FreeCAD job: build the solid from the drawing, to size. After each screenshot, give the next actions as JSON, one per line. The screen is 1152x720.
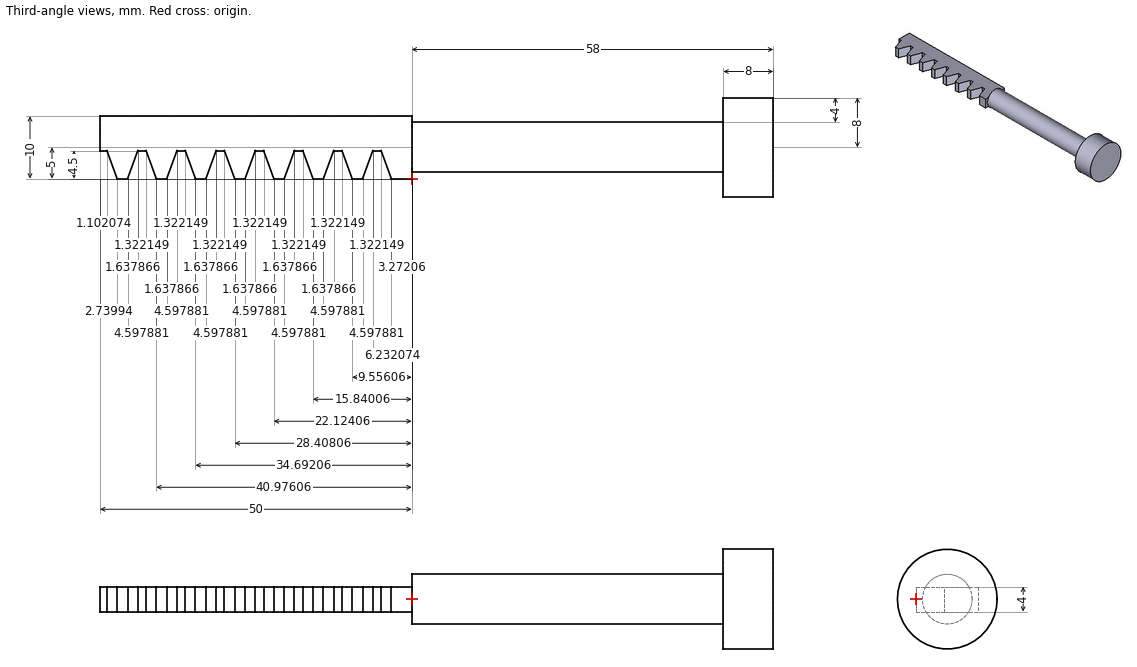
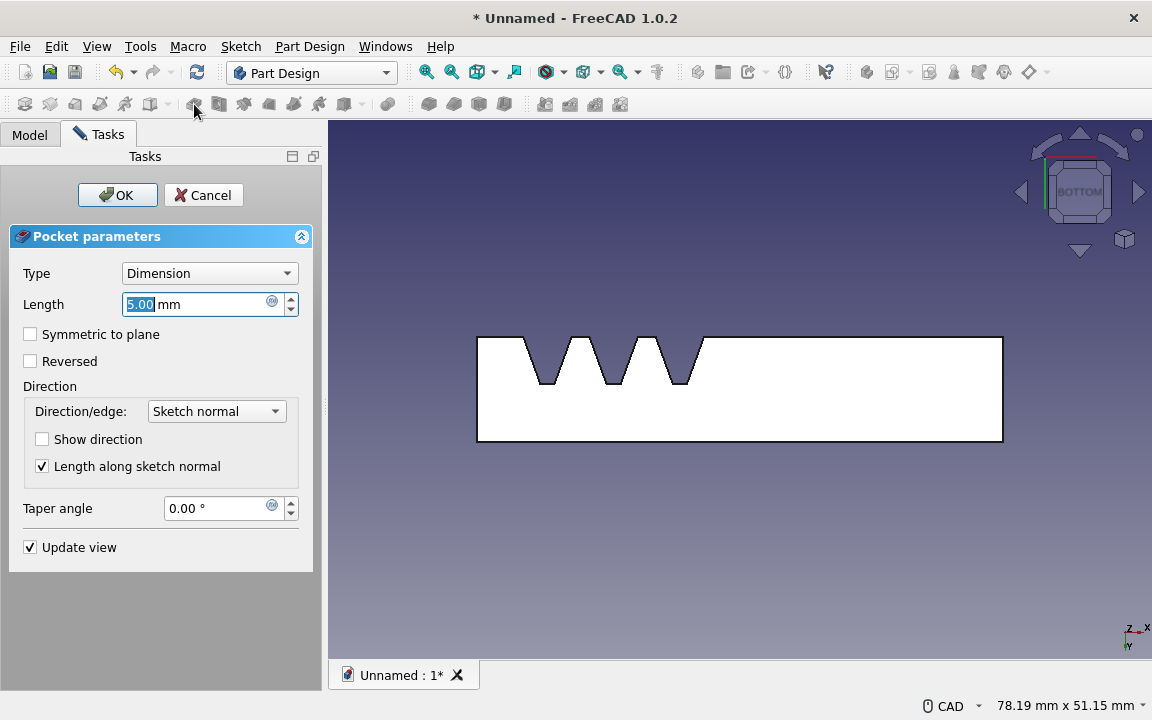
{"action": "left_click", "coordinate": [210, 274]}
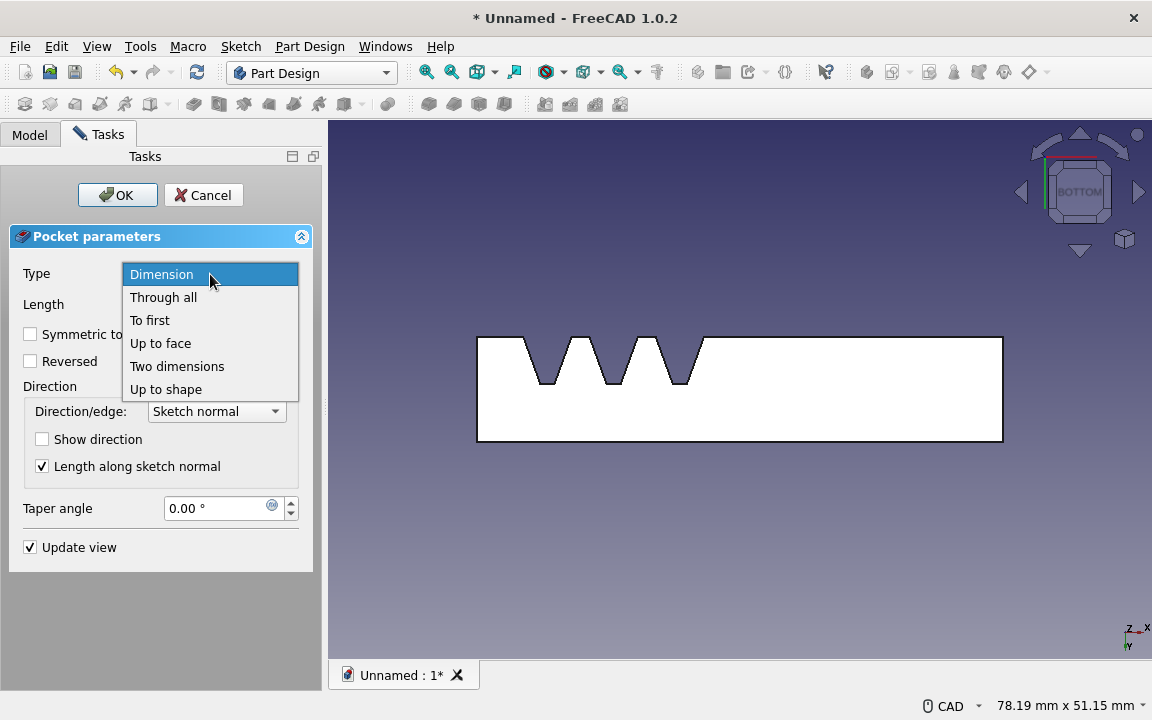
{"action": "left_click", "coordinate": [208, 298]}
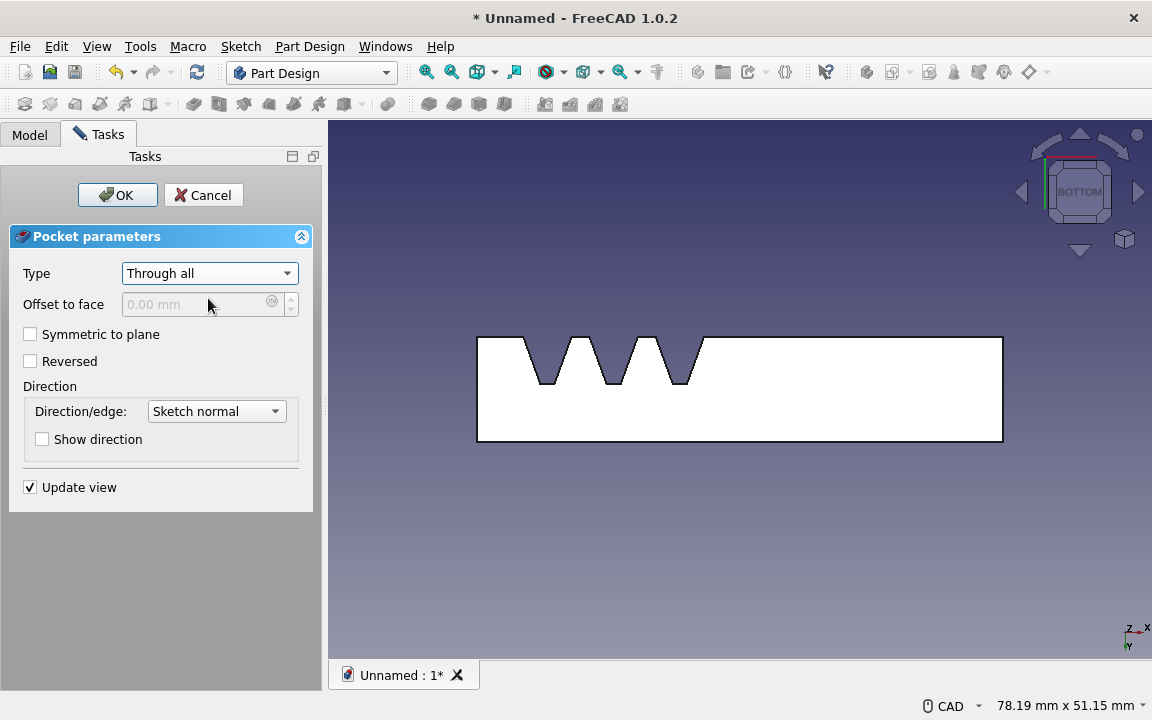
{"action": "left_click", "coordinate": [118, 195]}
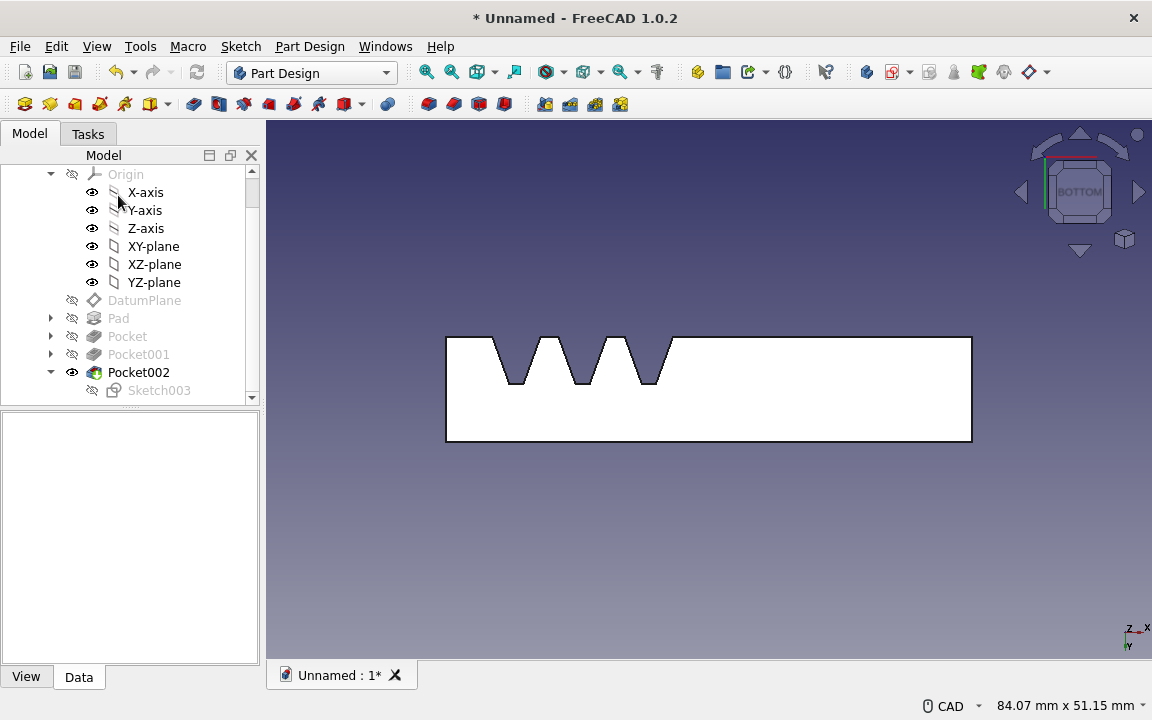
{"action": "left_click", "coordinate": [860, 389]}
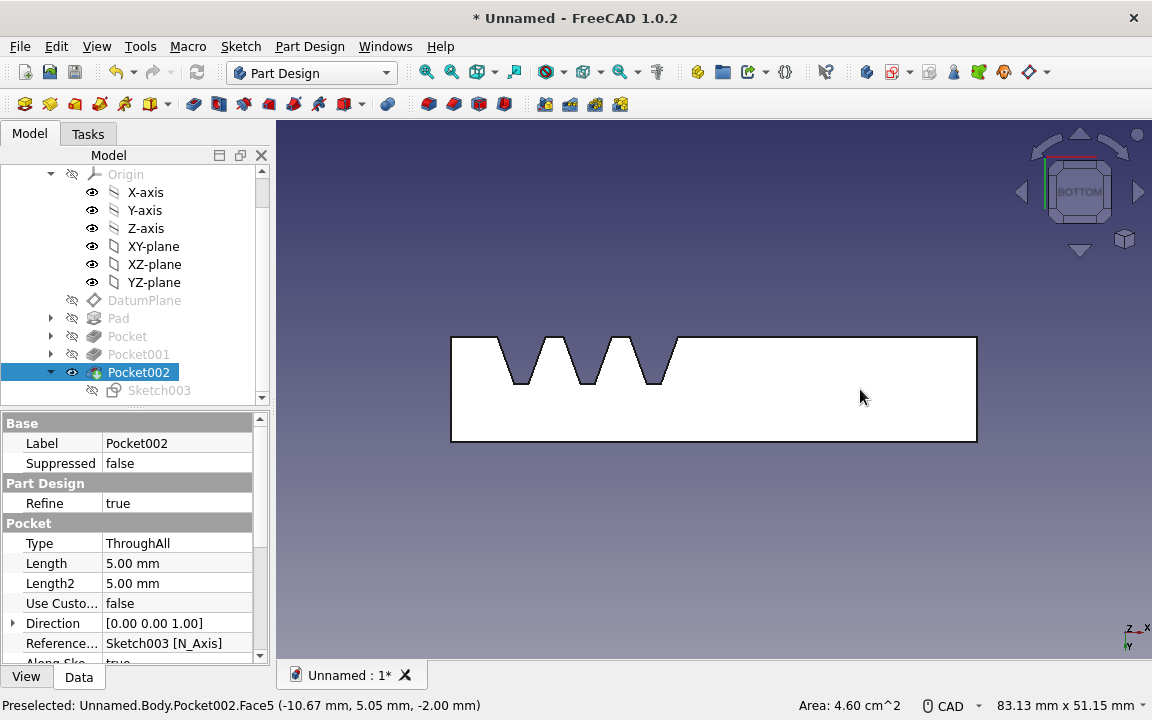
{"action": "left_click", "coordinate": [892, 72]}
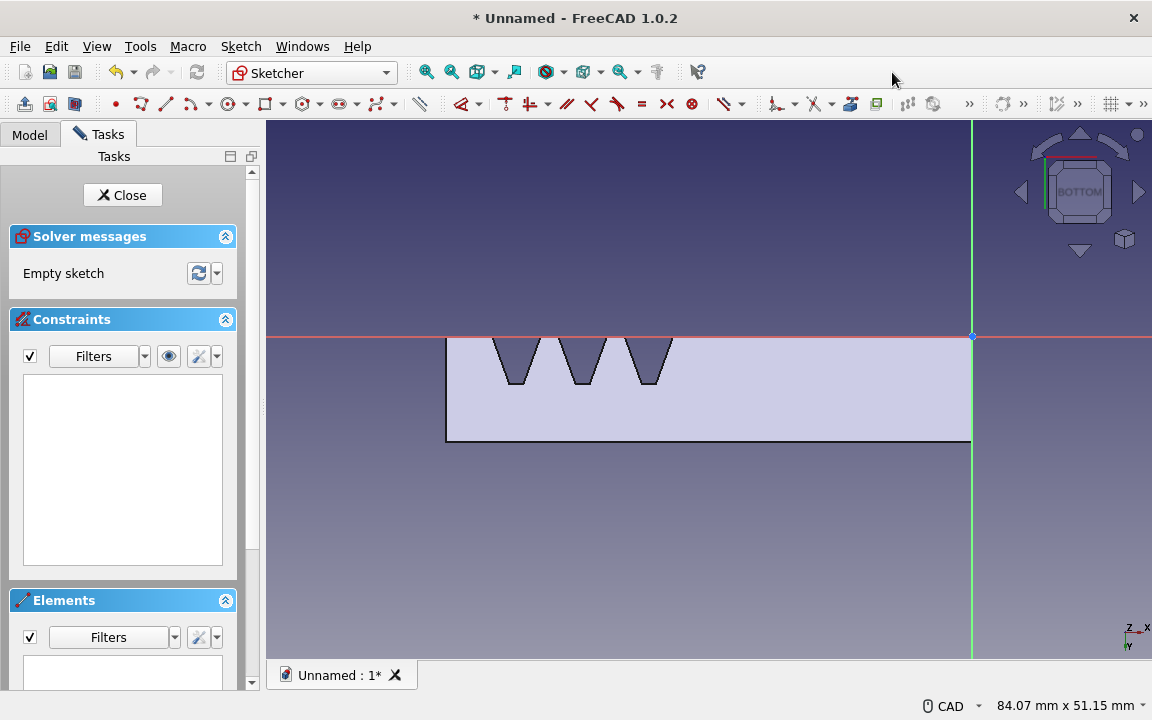
{"action": "scroll", "coordinate": [727, 356], "scroll_direction": "up", "scroll_amount": 10}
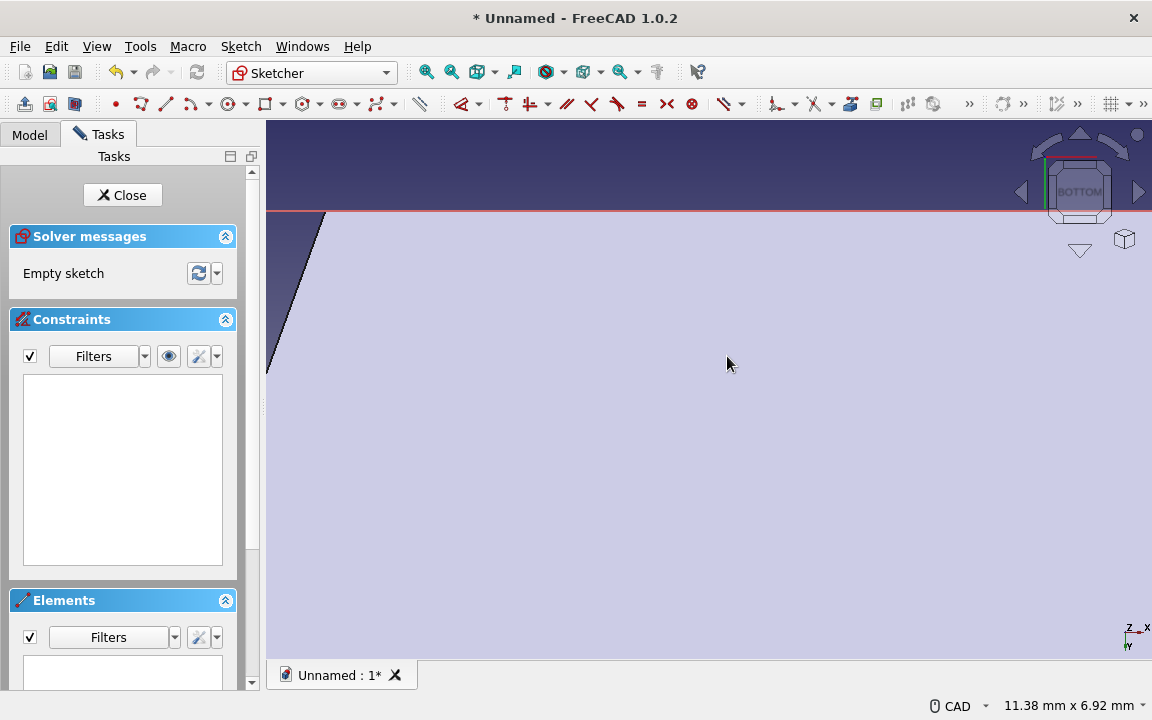
{"action": "left_click", "coordinate": [141, 104]}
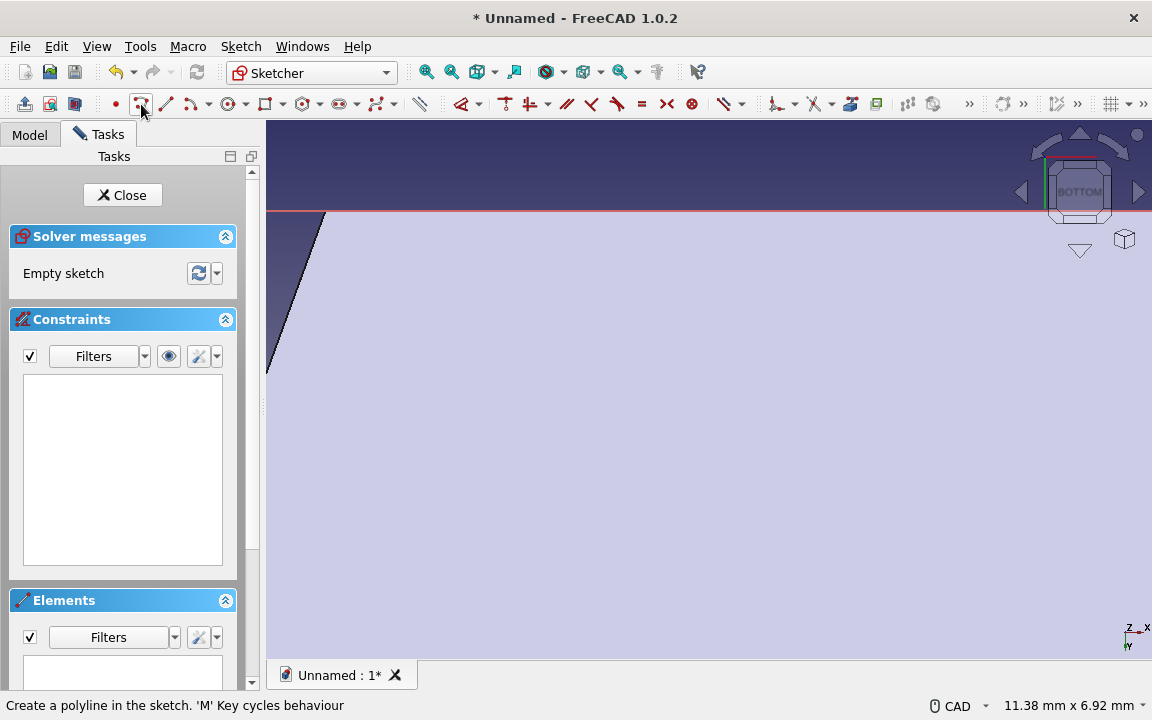
{"action": "left_click", "coordinate": [815, 211]}
{"action": "left_click", "coordinate": [457, 220]}
{"action": "left_click", "coordinate": [584, 562]}
{"action": "left_click", "coordinate": [687, 562]}
{"action": "left_click", "coordinate": [815, 211]}
{"action": "key", "text": "Escape"}
{"action": "key", "text": "Escape"}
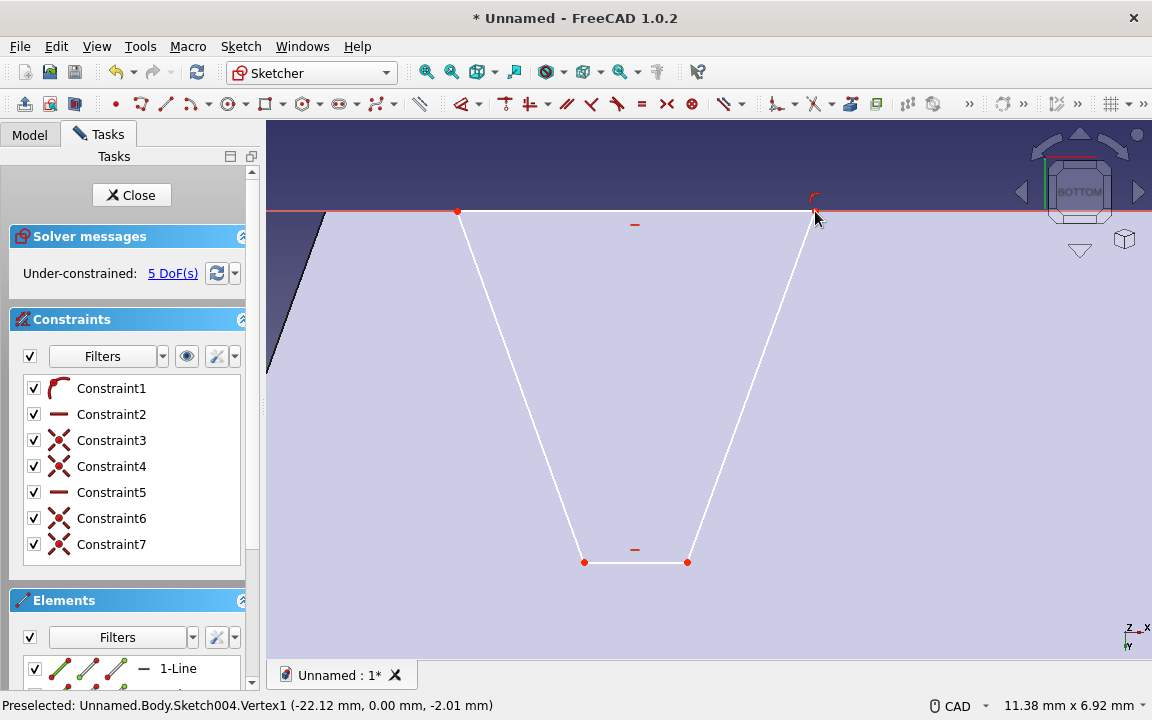
{"action": "left_click", "coordinate": [460, 104]}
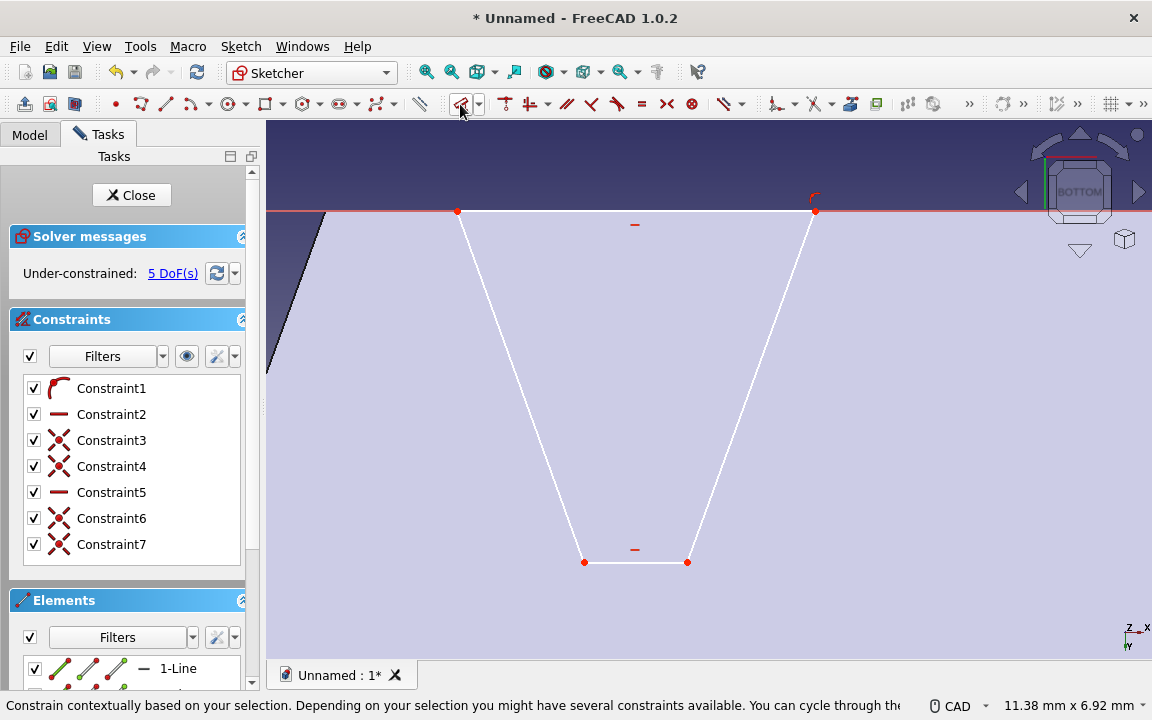
{"action": "left_click", "coordinate": [584, 563]}
{"action": "left_click", "coordinate": [550, 387]}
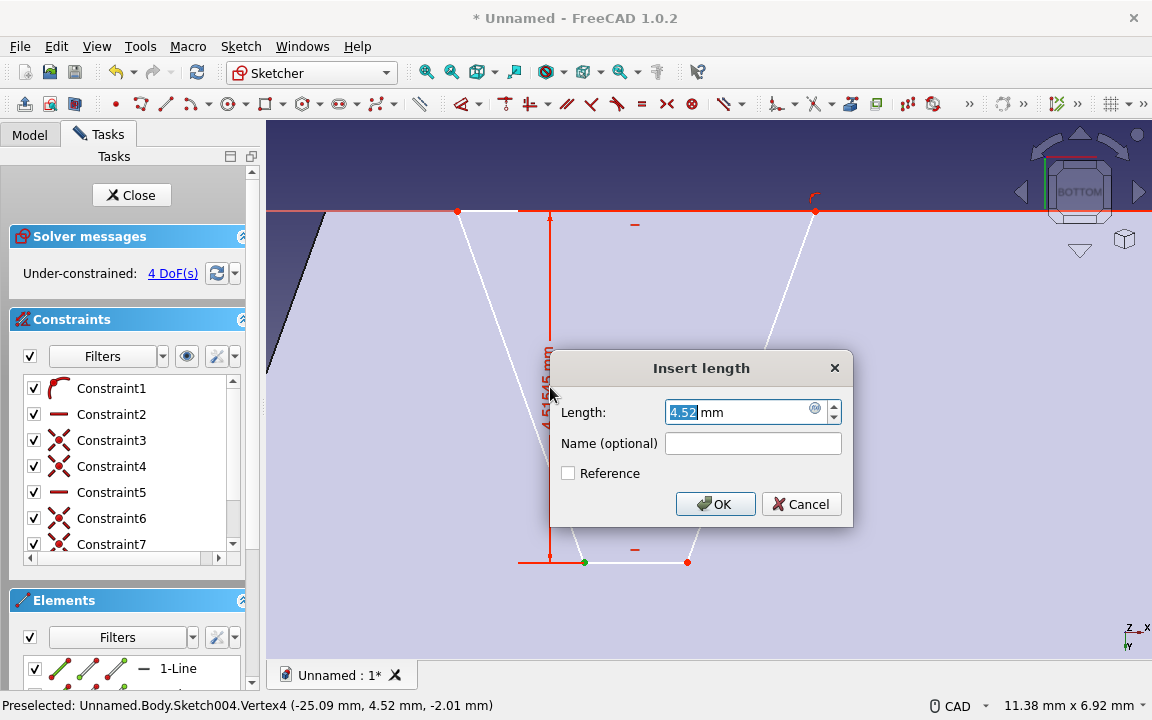
{"action": "type", "text": "4.5"}
{"action": "key", "text": "Return"}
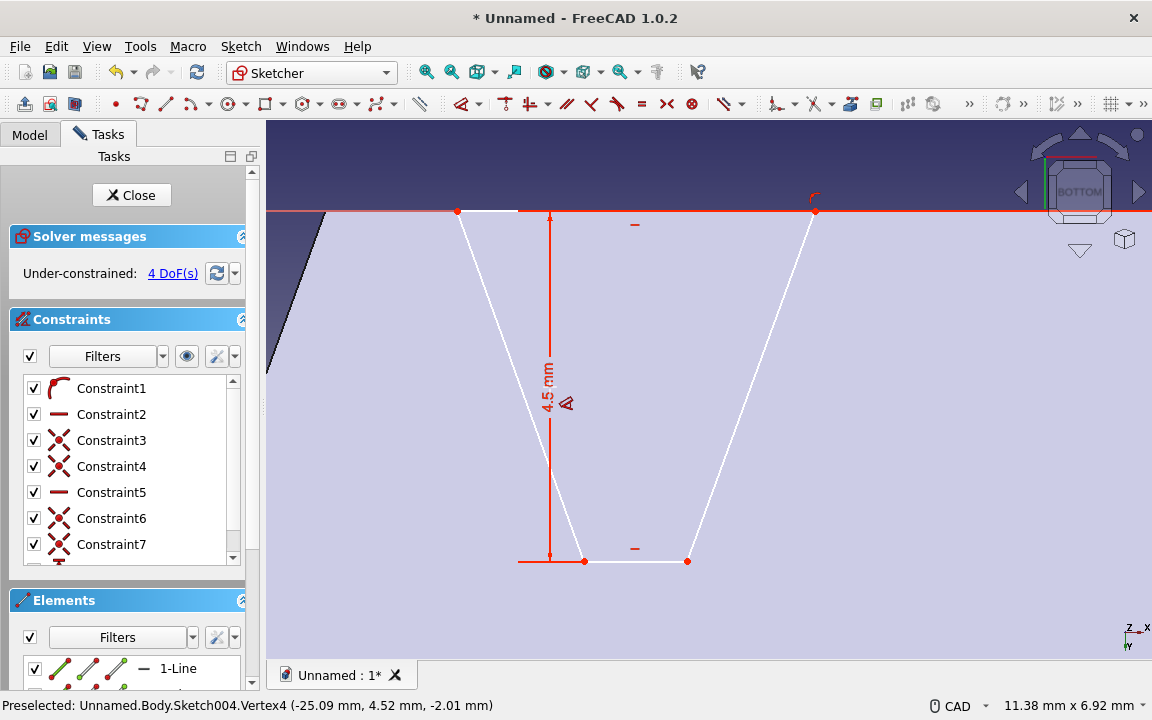
{"action": "left_click", "coordinate": [708, 211]}
{"action": "left_click", "coordinate": [636, 177]}